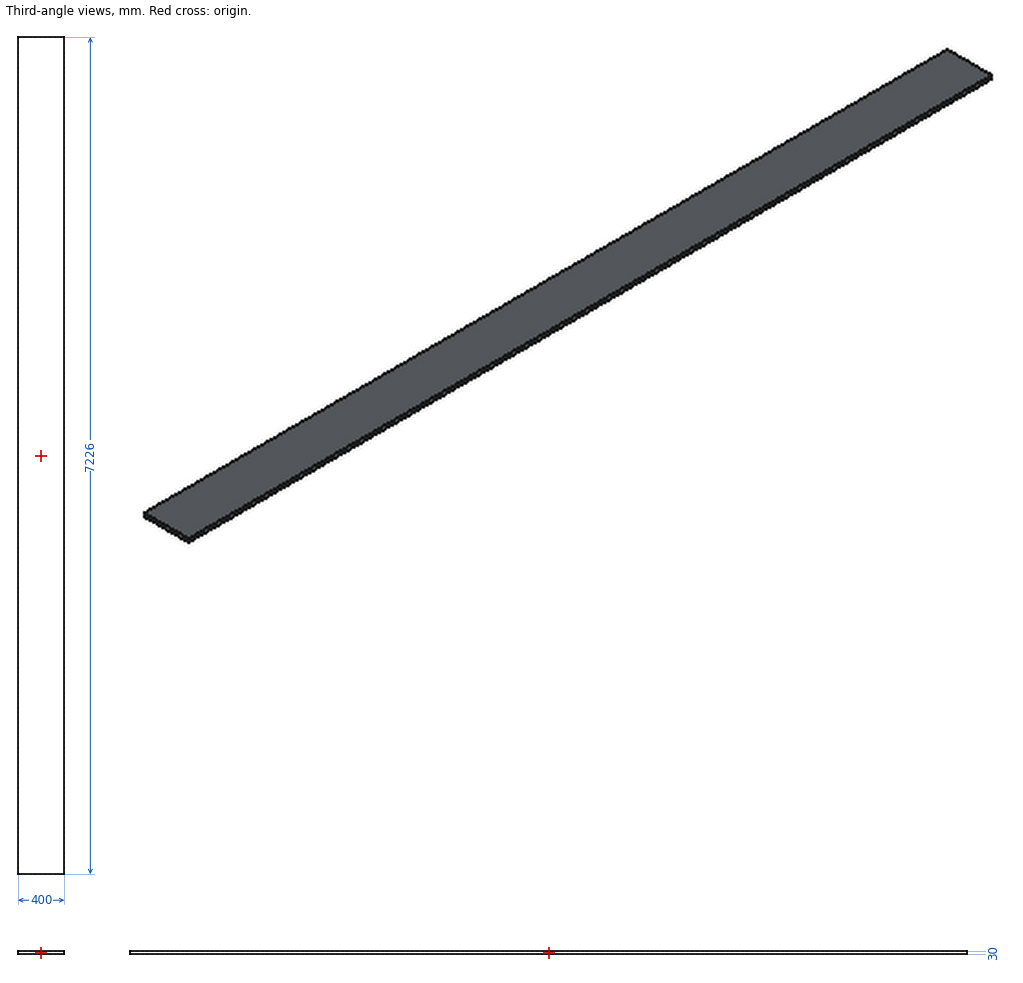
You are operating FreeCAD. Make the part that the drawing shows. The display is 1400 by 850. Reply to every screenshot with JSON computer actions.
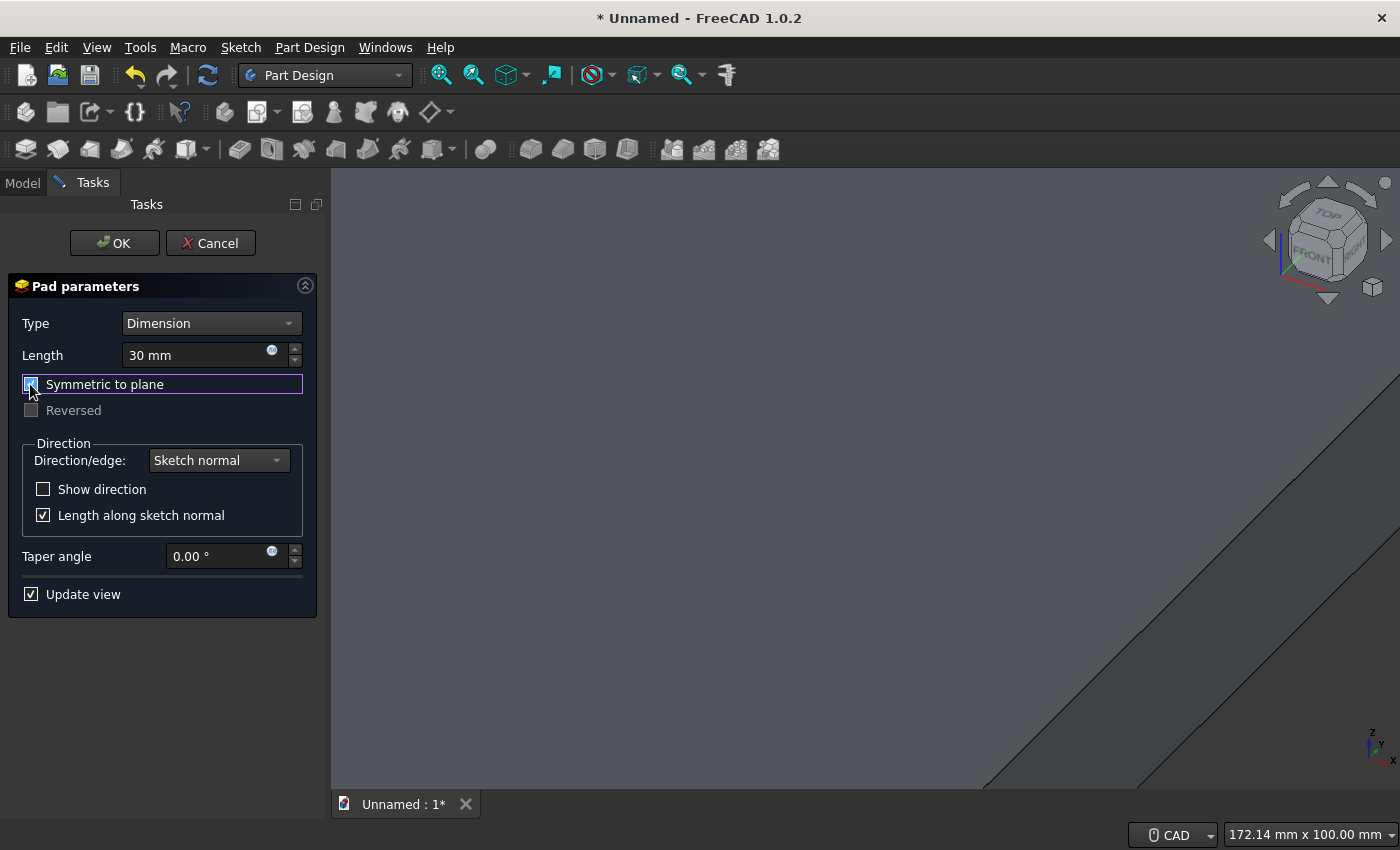
{"action": "left_click", "coordinate": [115, 243]}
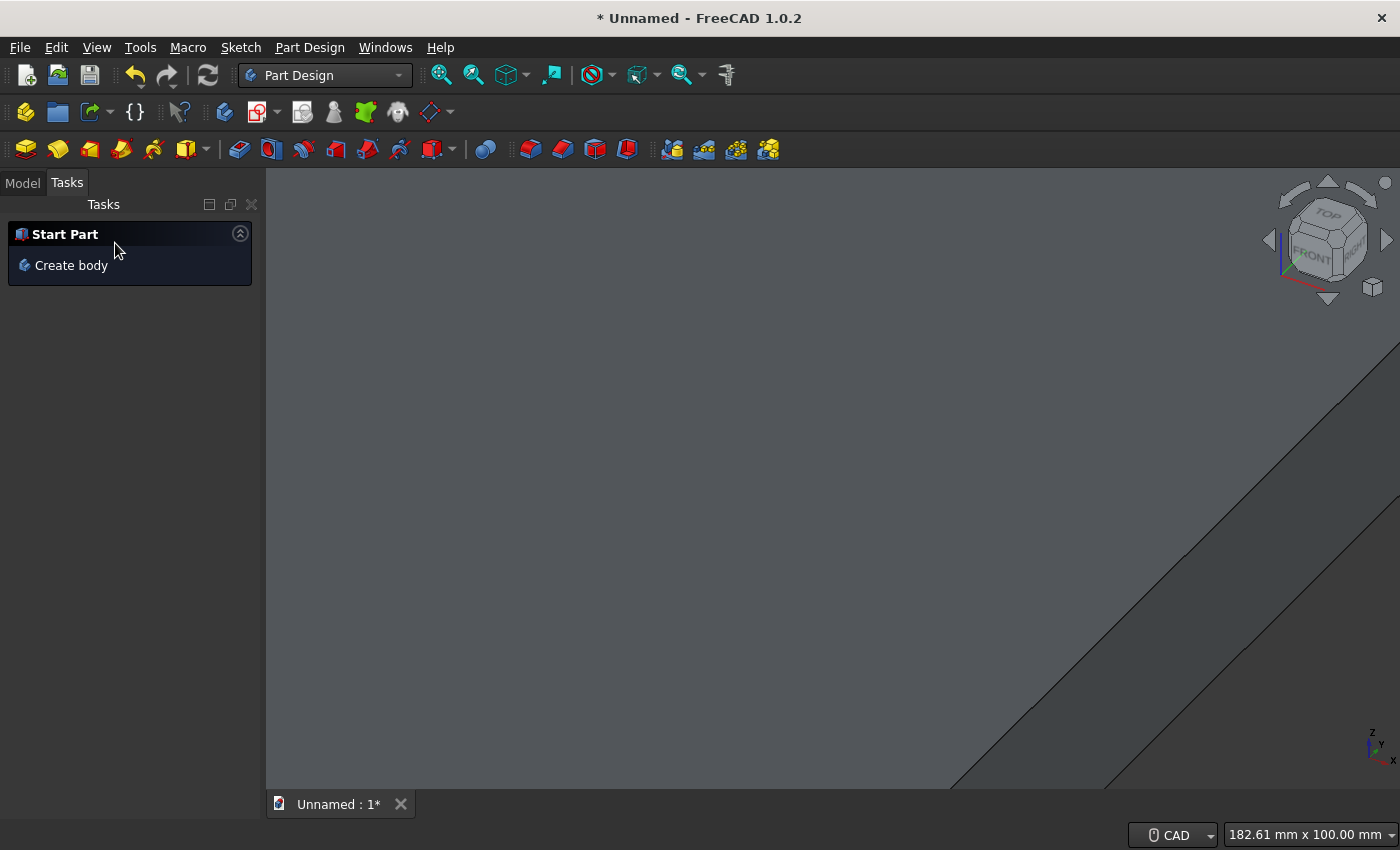
{"action": "key", "text": "0"}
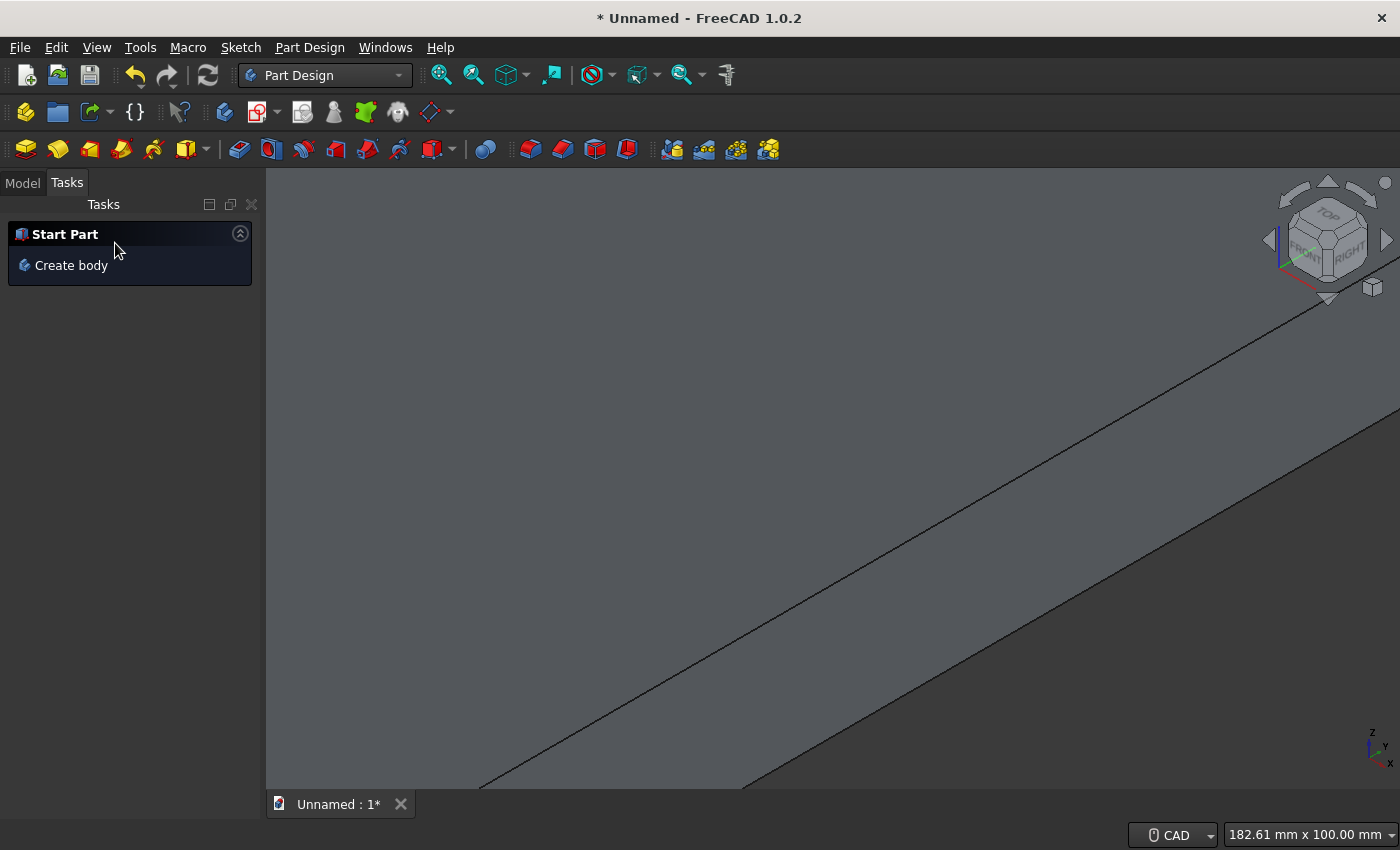
{"action": "left_click", "coordinate": [442, 76]}